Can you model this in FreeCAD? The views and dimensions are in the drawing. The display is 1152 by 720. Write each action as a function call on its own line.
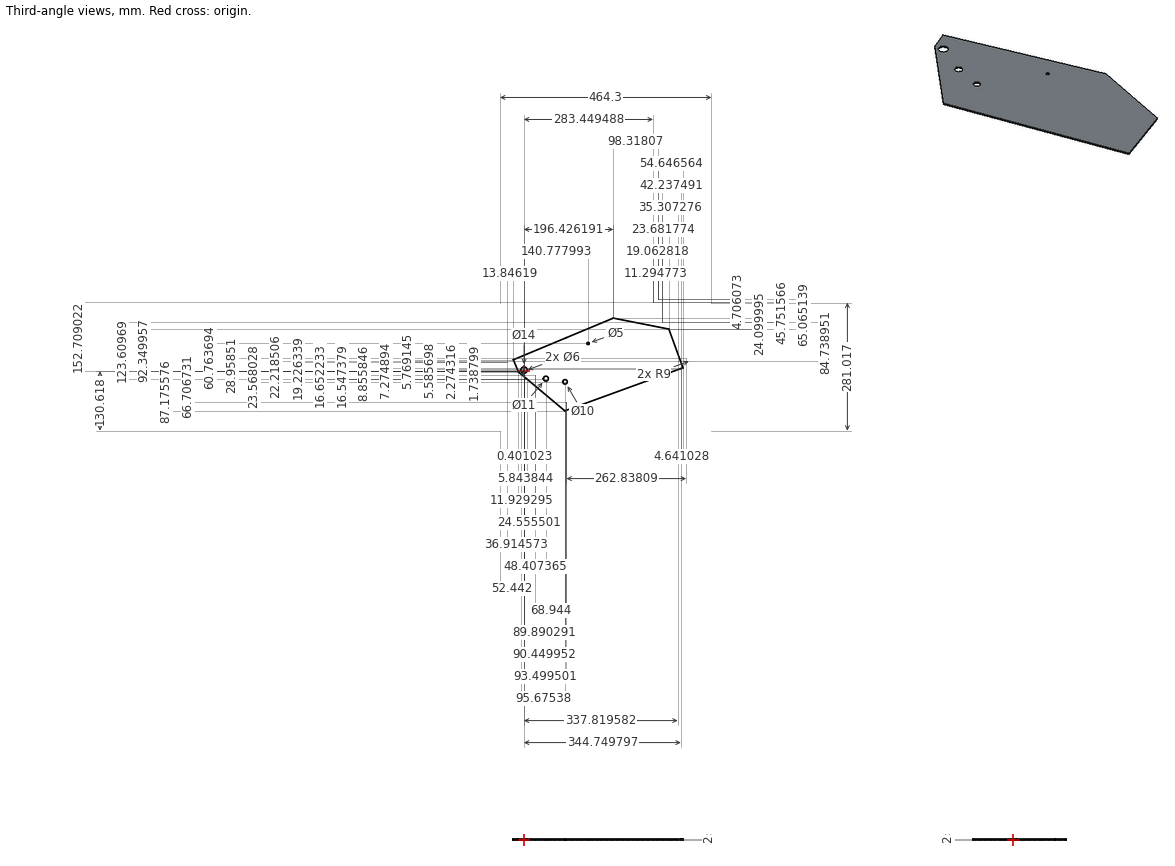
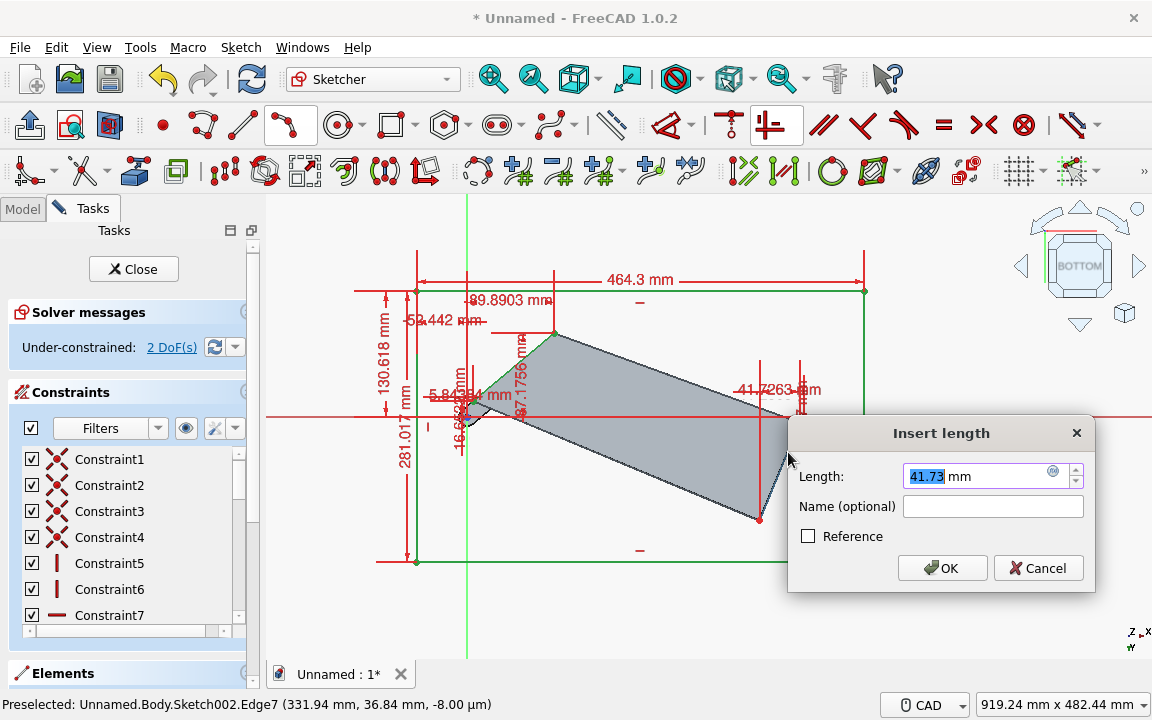
text(42.237491)
key(Return)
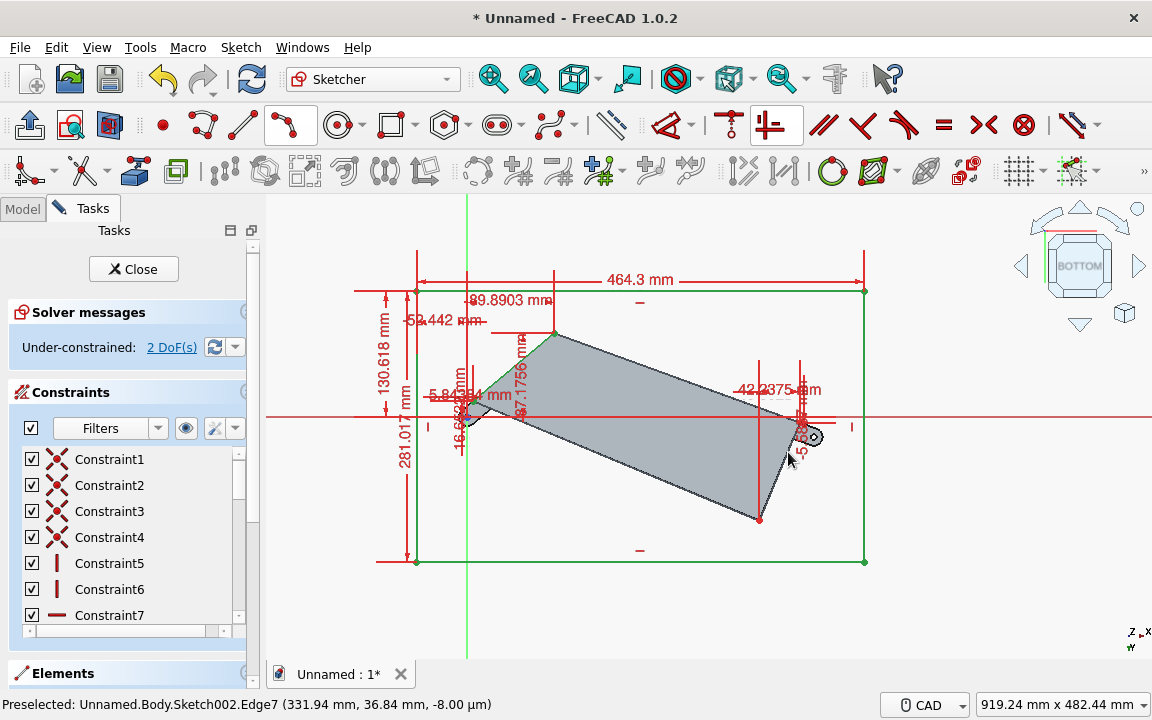
click(674, 485)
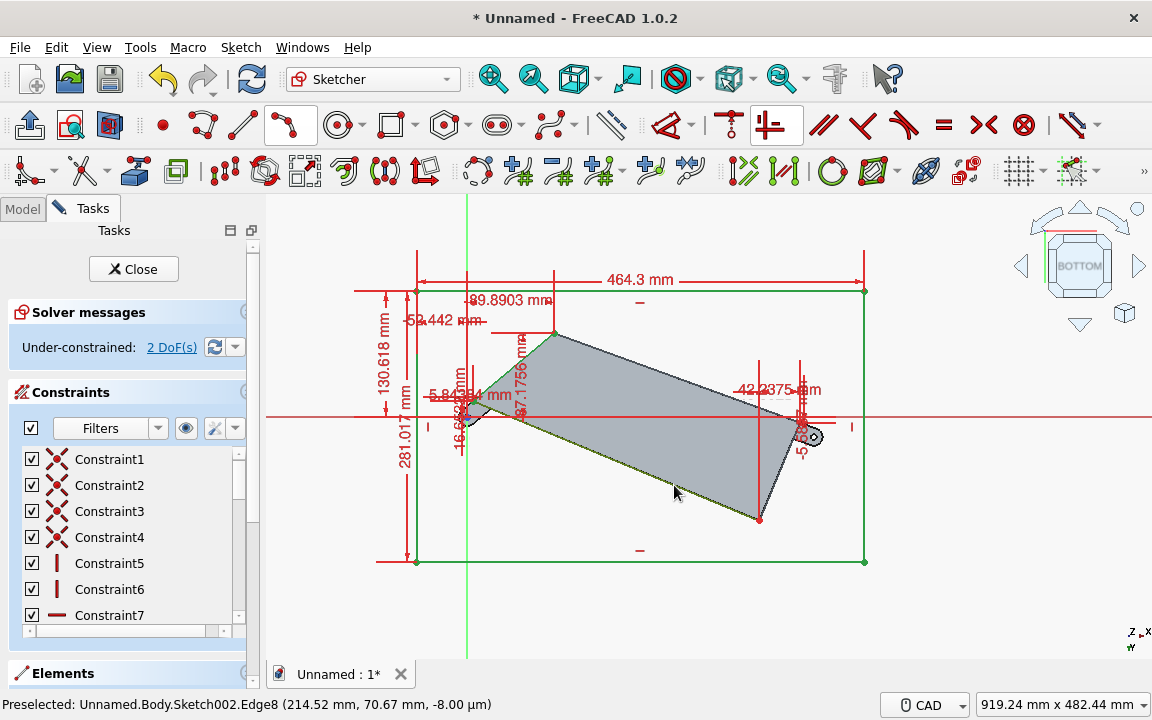
key(i)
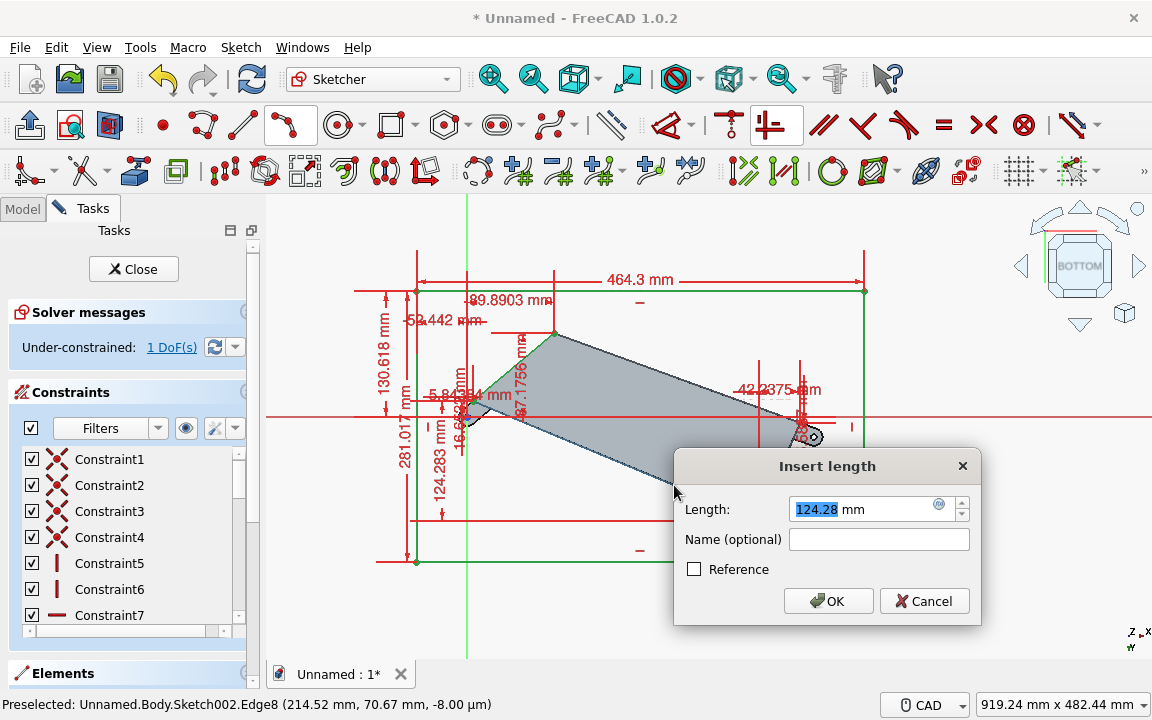
text(123.60969)
key(Return)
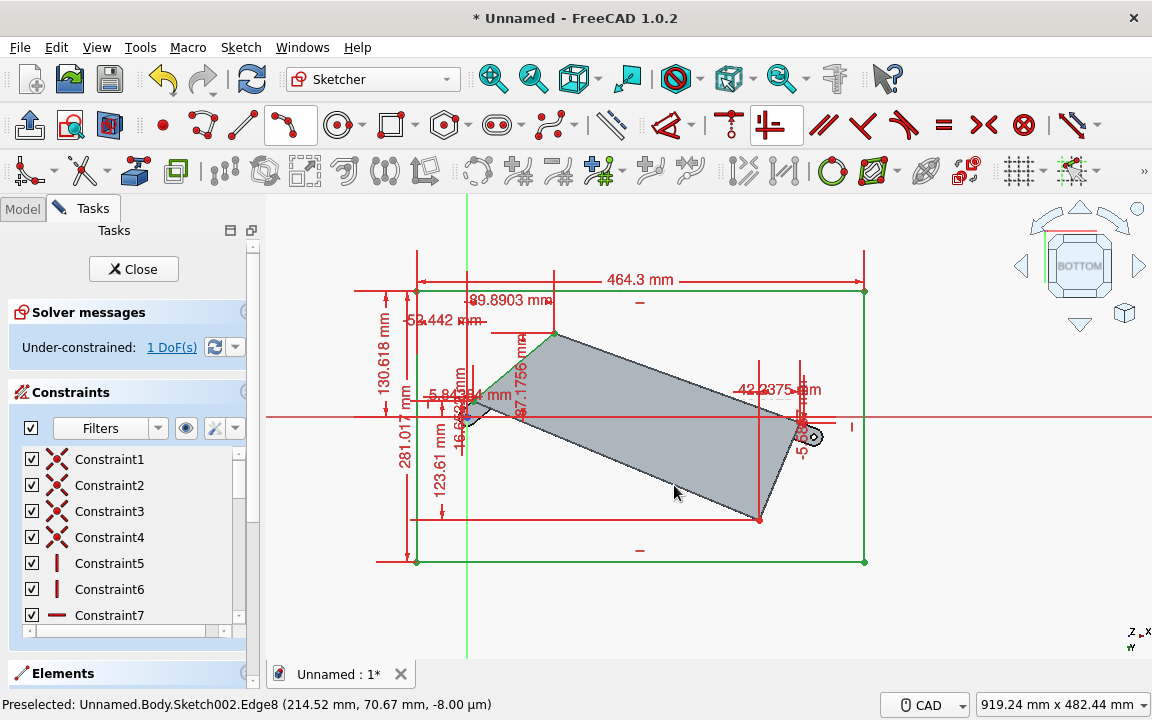
click(800, 423)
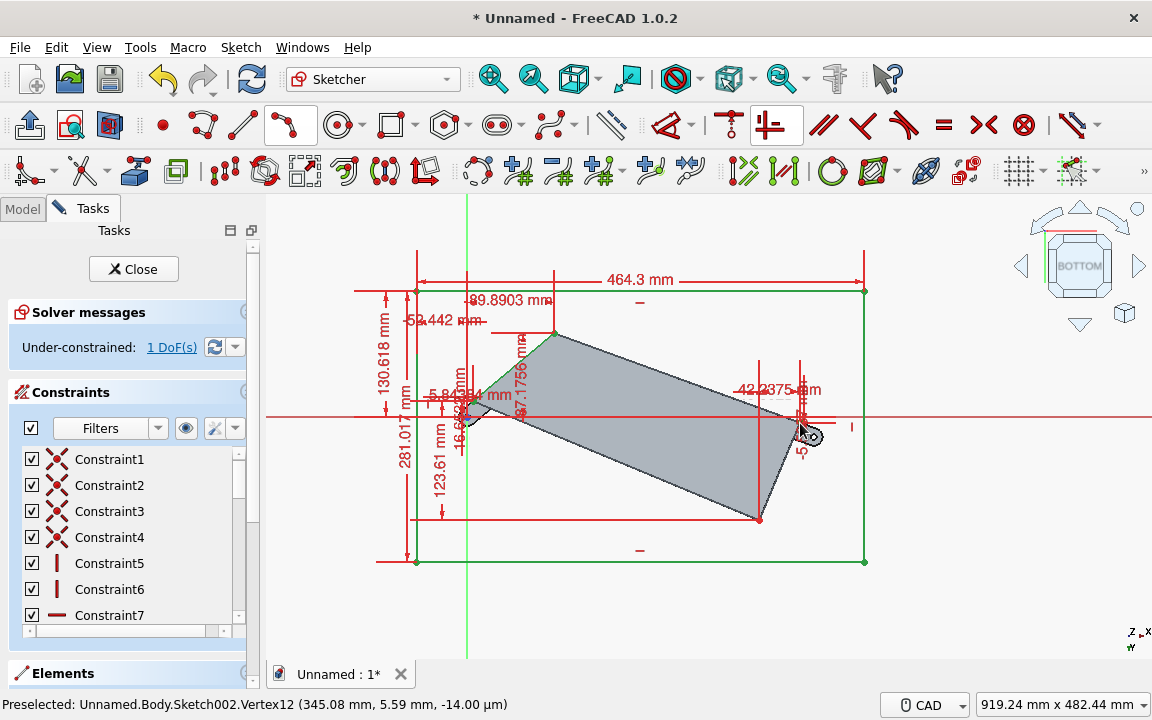
click(694, 126)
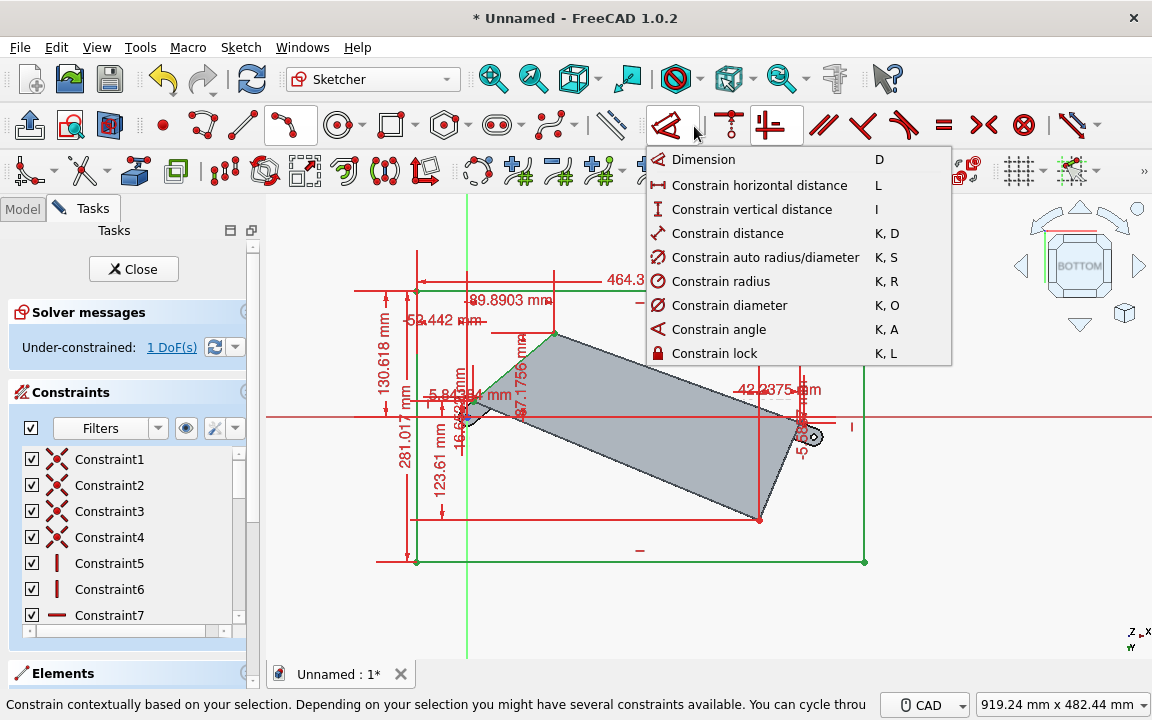
click(799, 185)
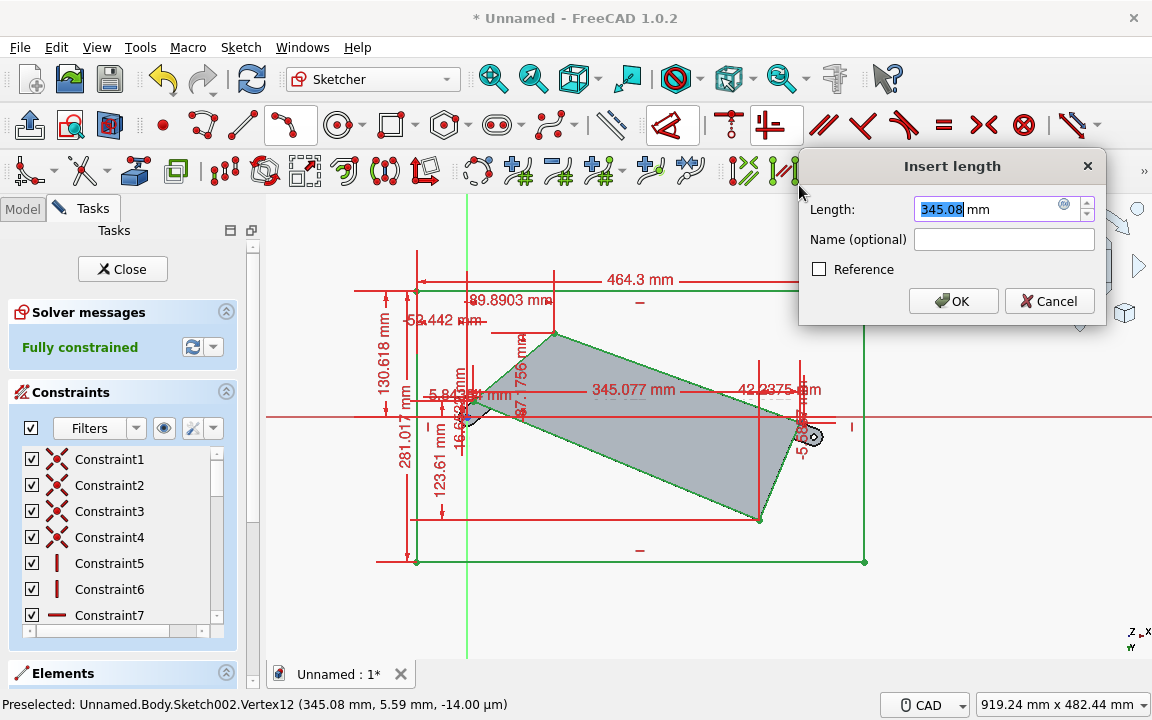
text(344.749797)
key(Return)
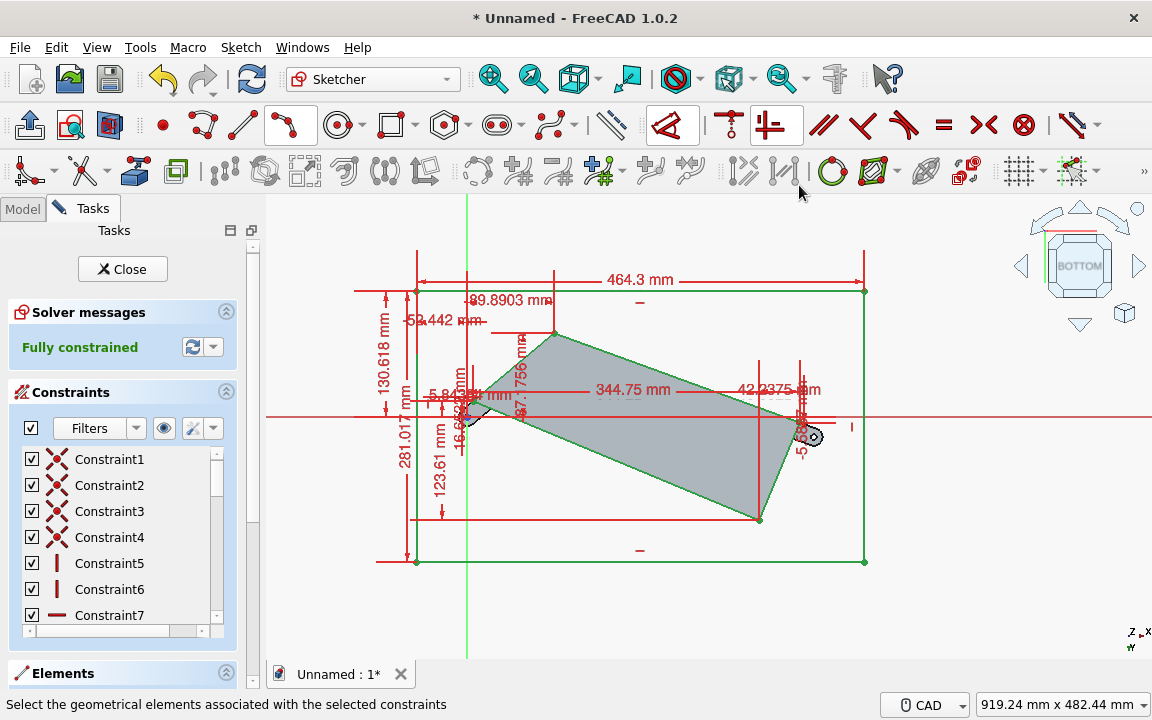
click(123, 269)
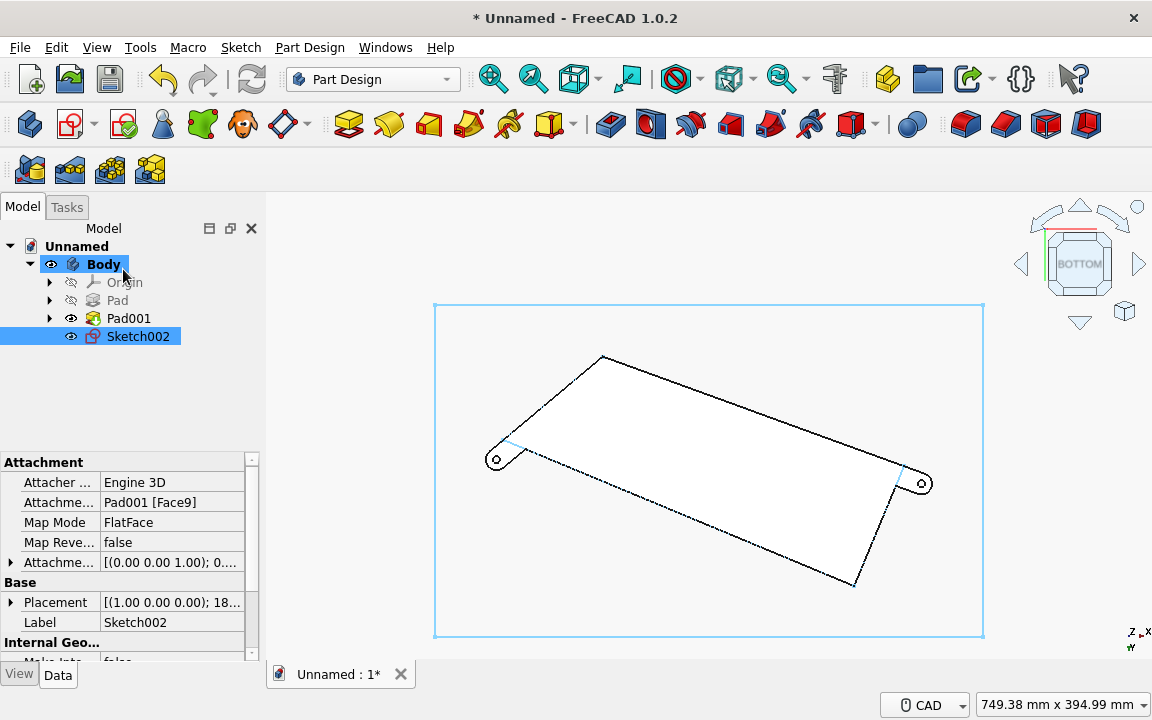
click(612, 124)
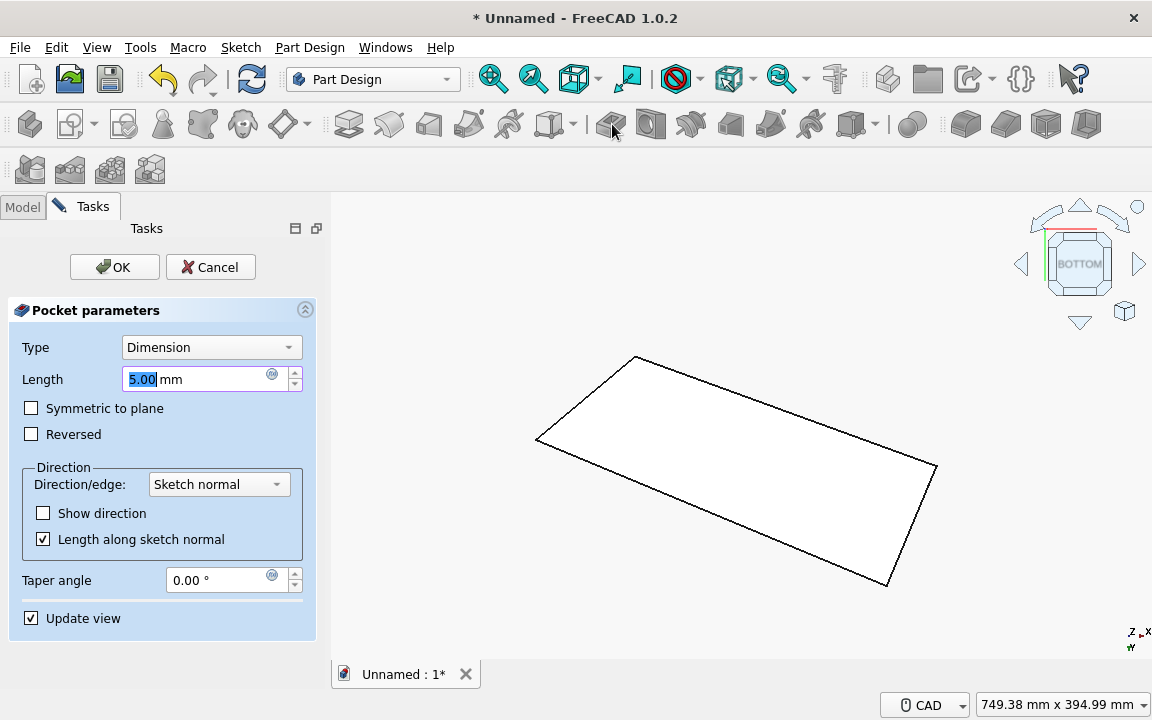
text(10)
key(Tab)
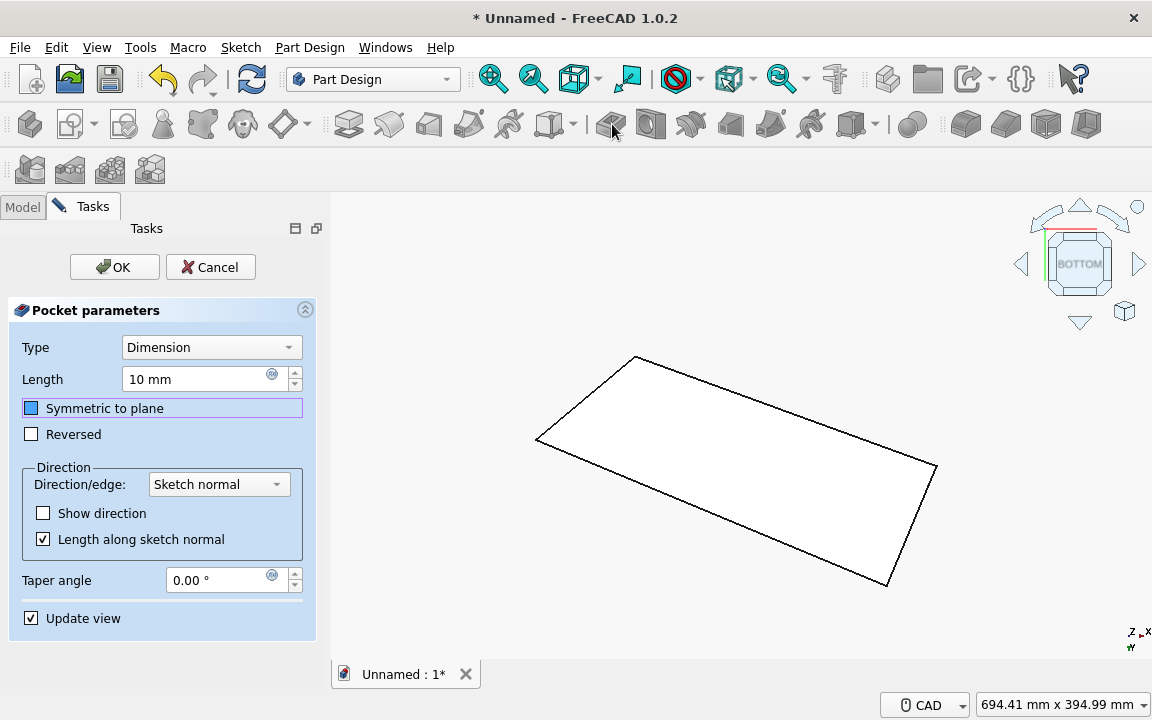
click(115, 267)